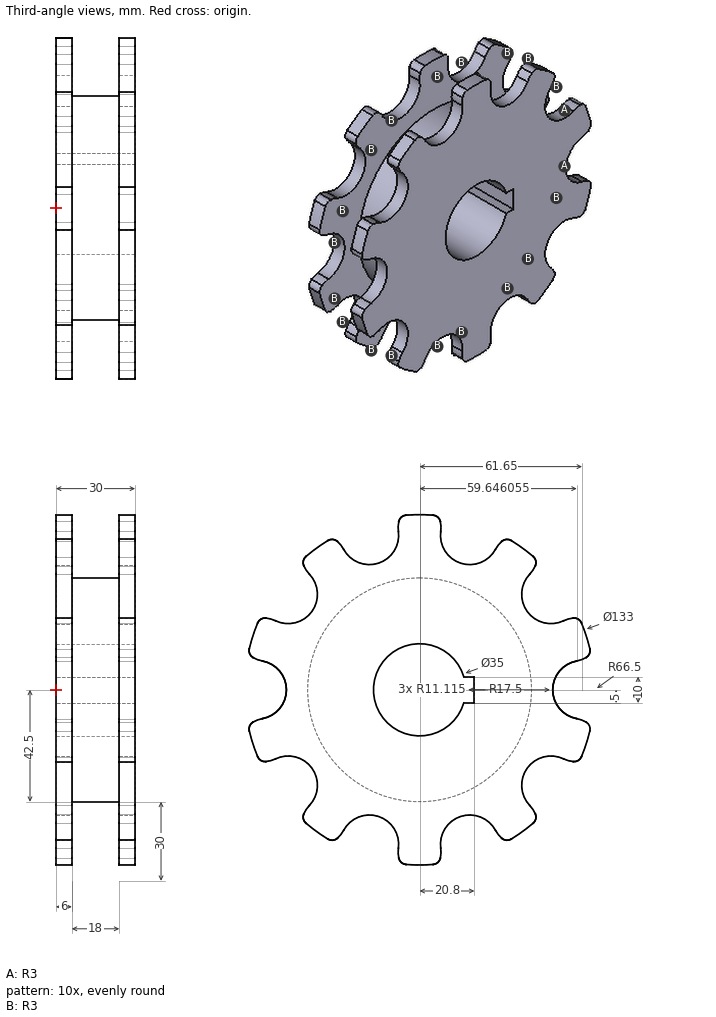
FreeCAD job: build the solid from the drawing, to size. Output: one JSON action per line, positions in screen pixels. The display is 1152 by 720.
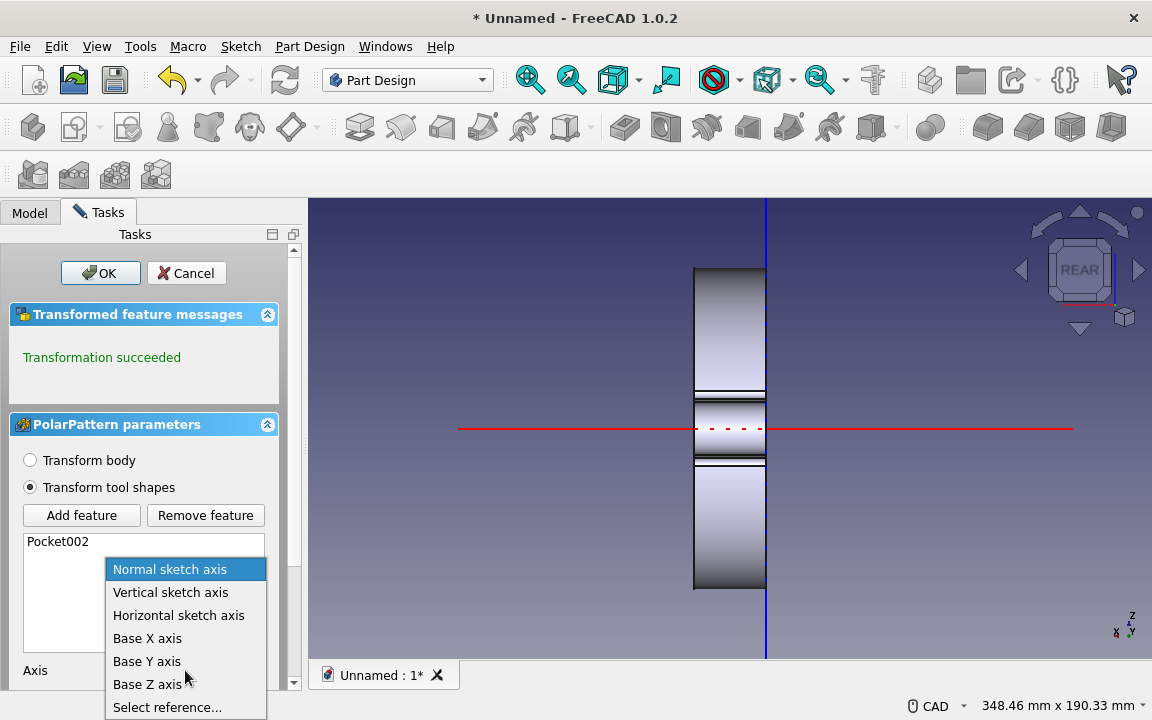
{"action": "left_click", "coordinate": [184, 638]}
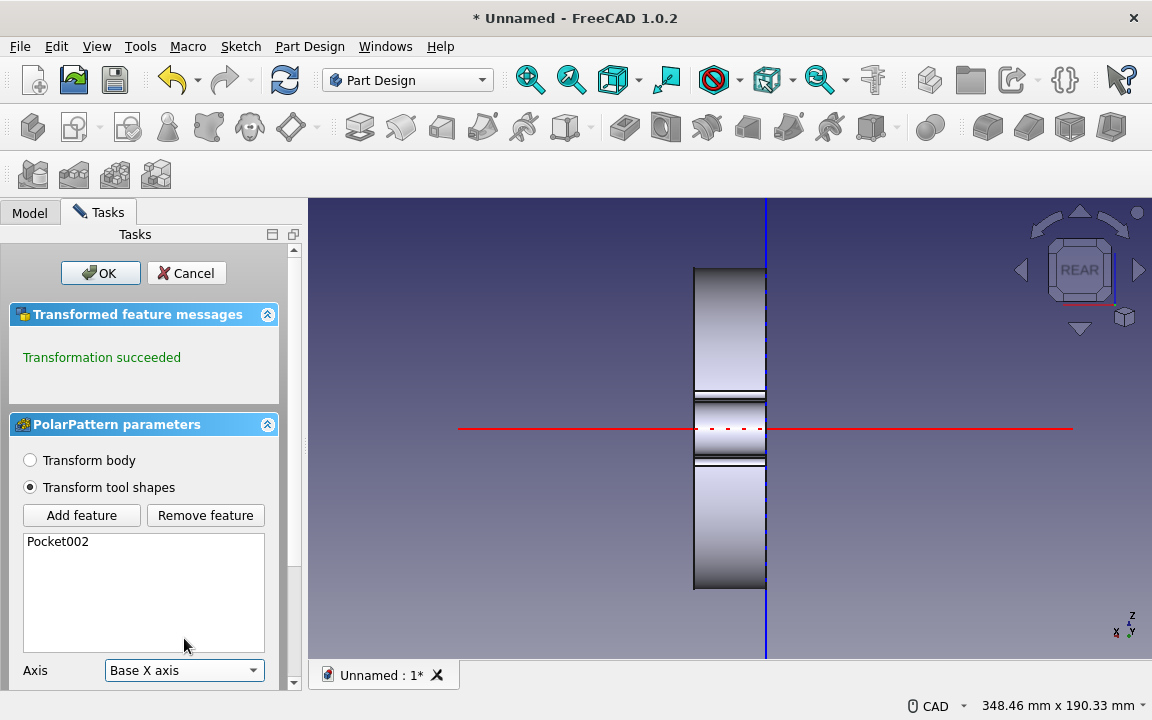
{"action": "scroll", "coordinate": [294, 467], "scroll_direction": "down", "scroll_amount": 3}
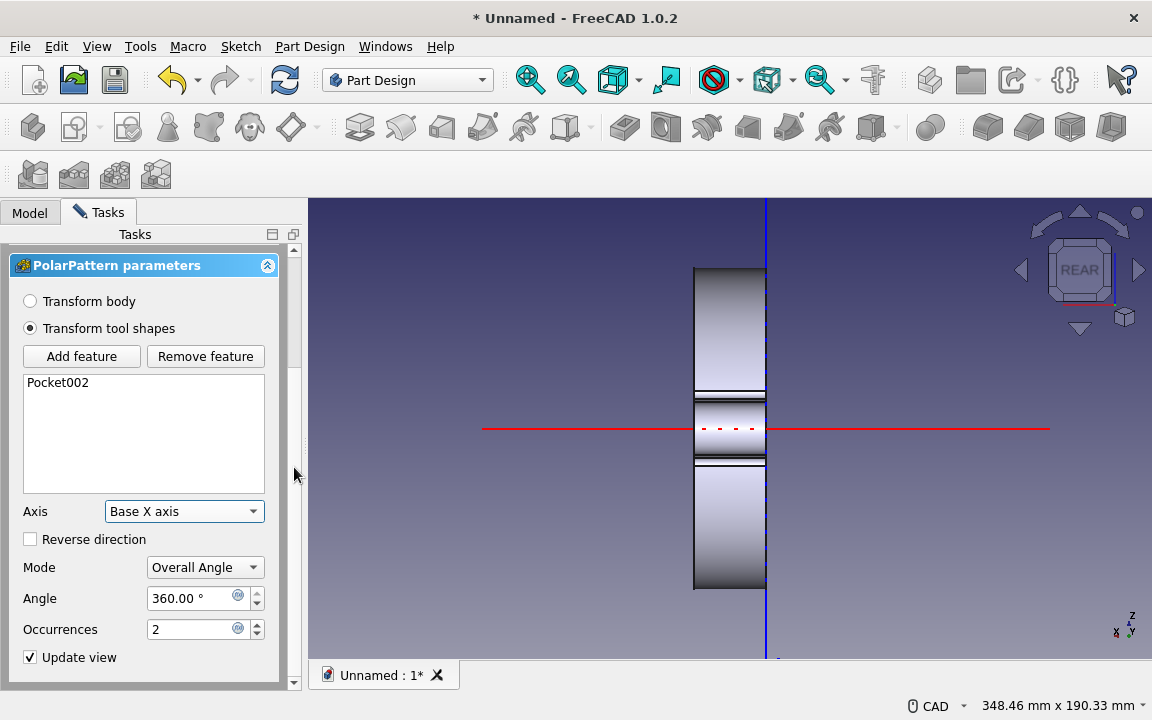
{"action": "triple_click", "coordinate": [199, 630]}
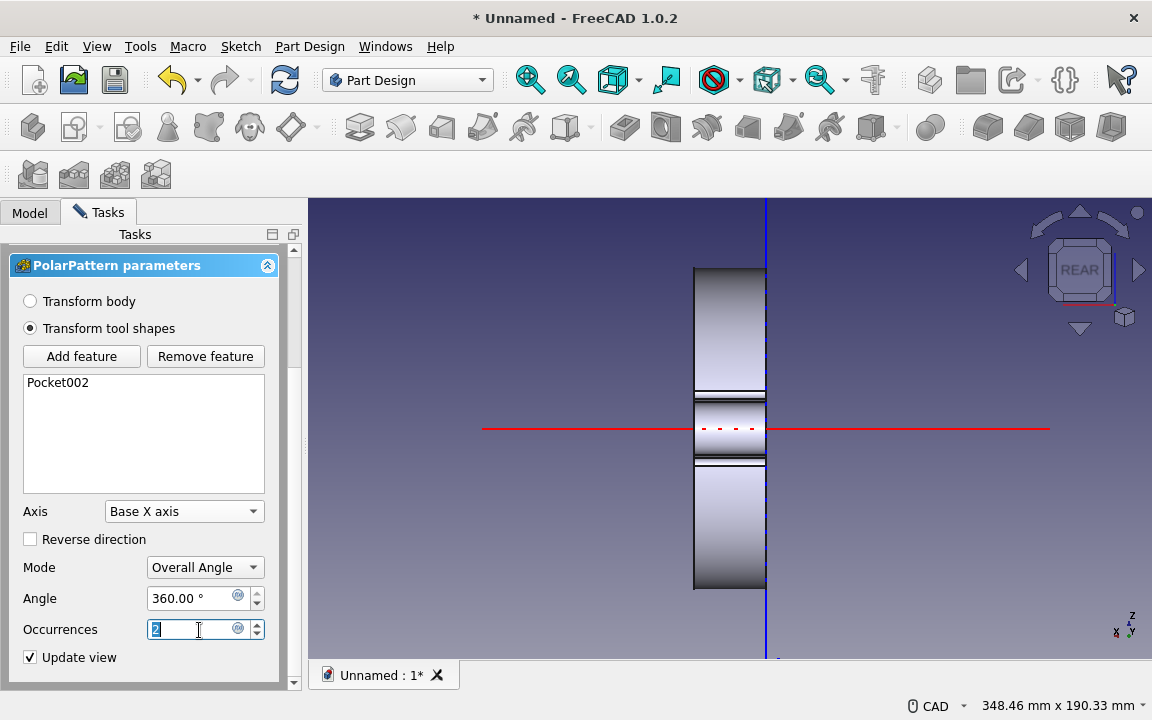
{"action": "type", "text": "10"}
{"action": "key", "text": "Tab"}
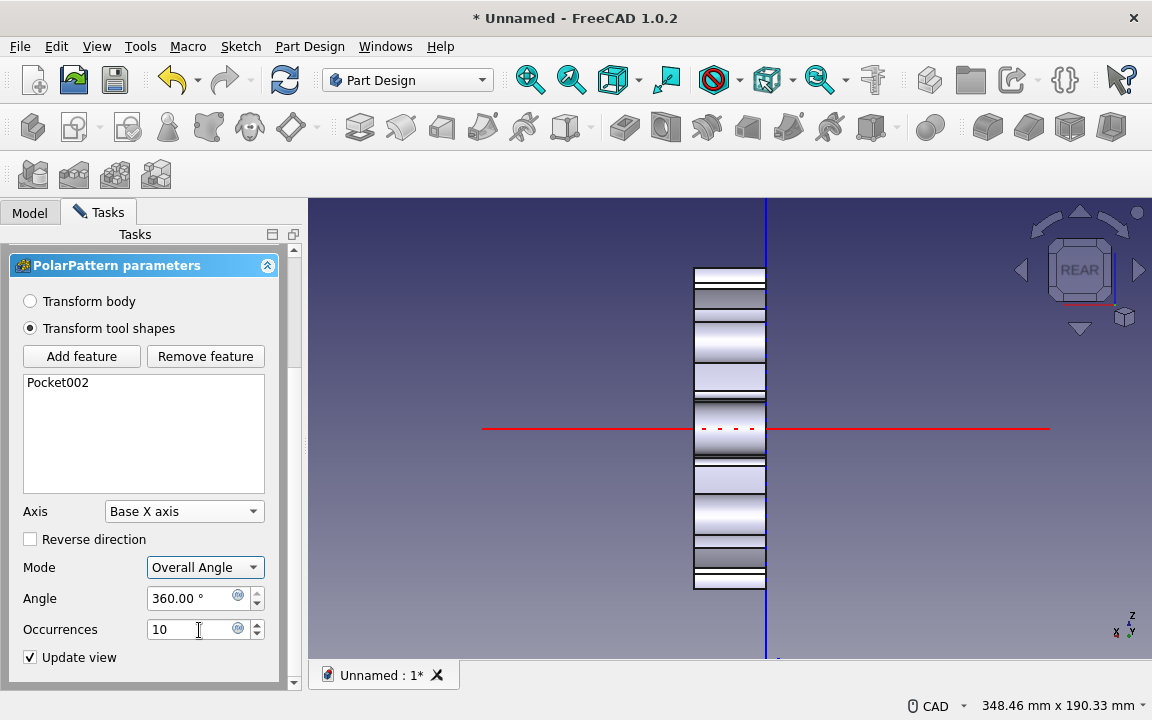
{"action": "scroll", "coordinate": [294, 467], "scroll_direction": "up", "scroll_amount": 4}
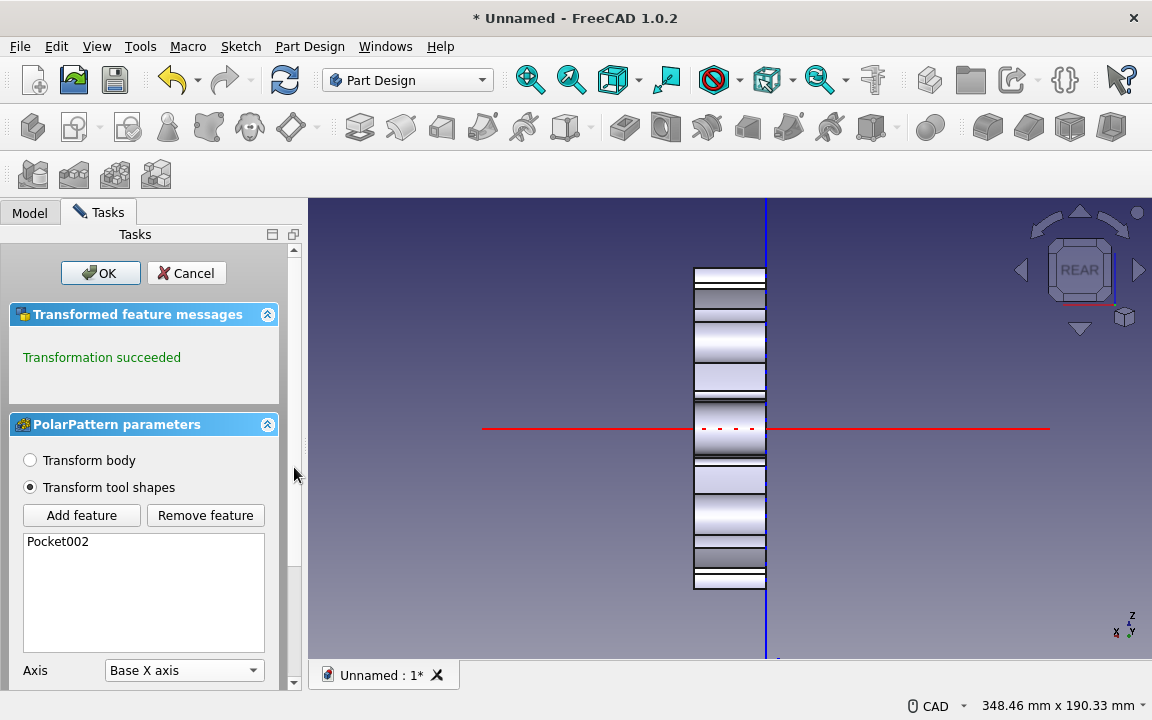
{"action": "left_click", "coordinate": [101, 273]}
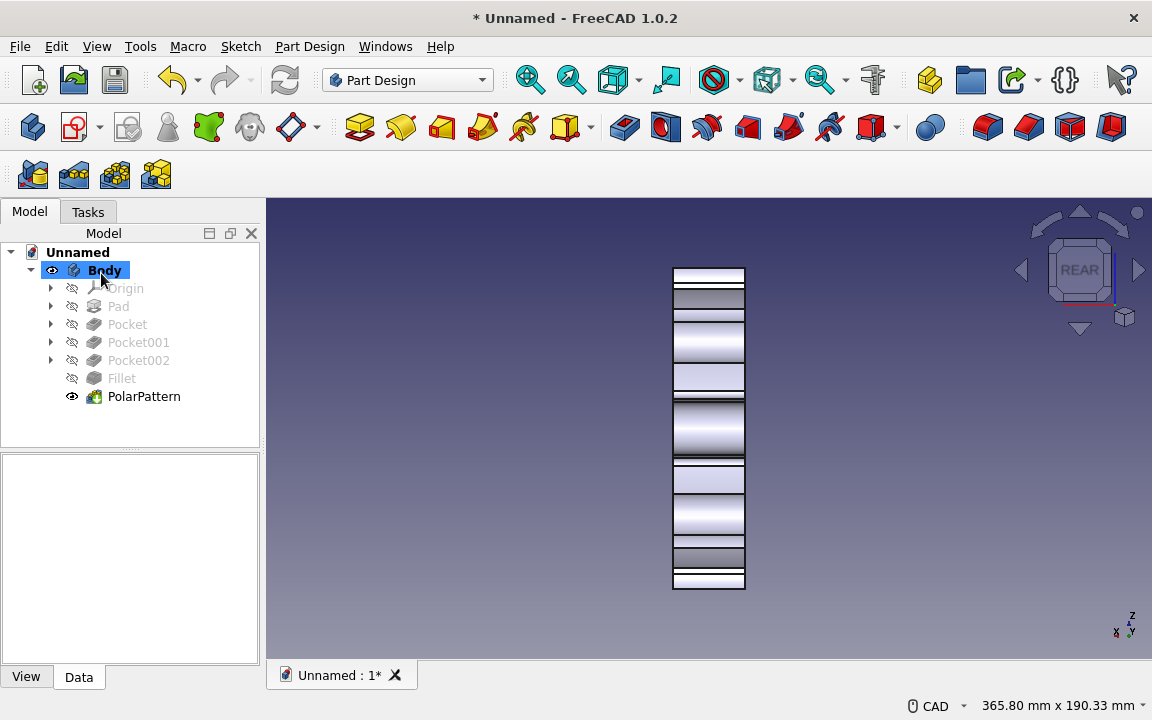
{"action": "left_click", "coordinate": [709, 308]}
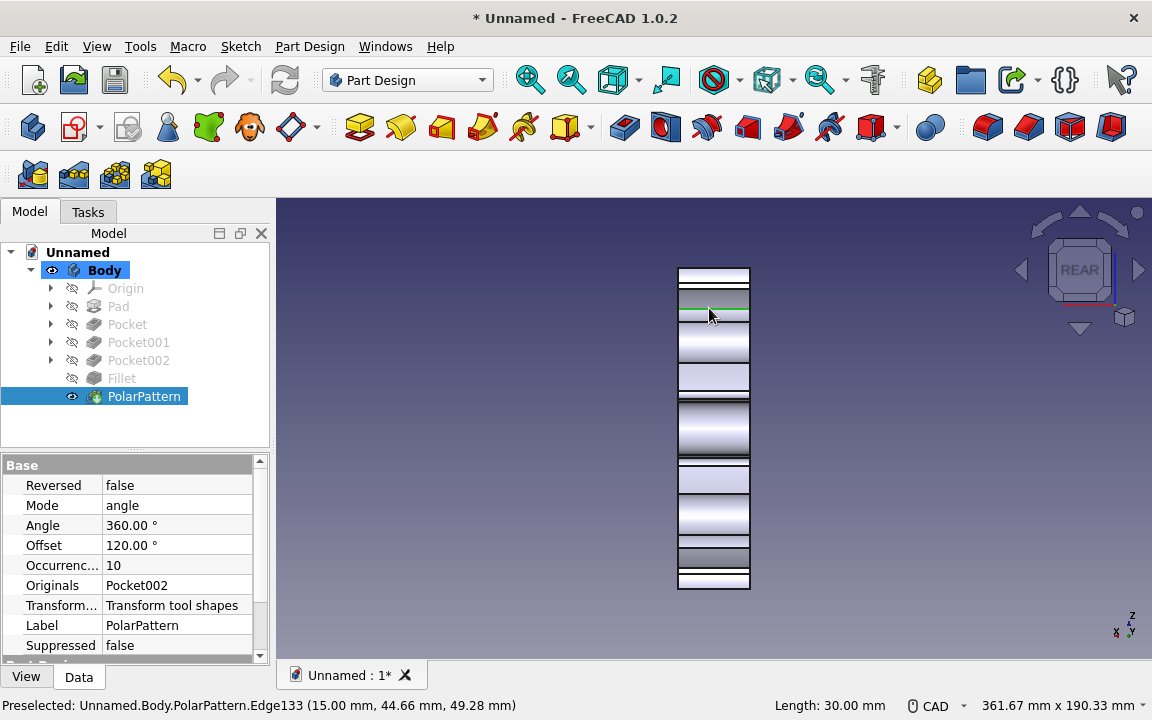
{"action": "left_click", "coordinate": [714, 547], "text": "ctrl"}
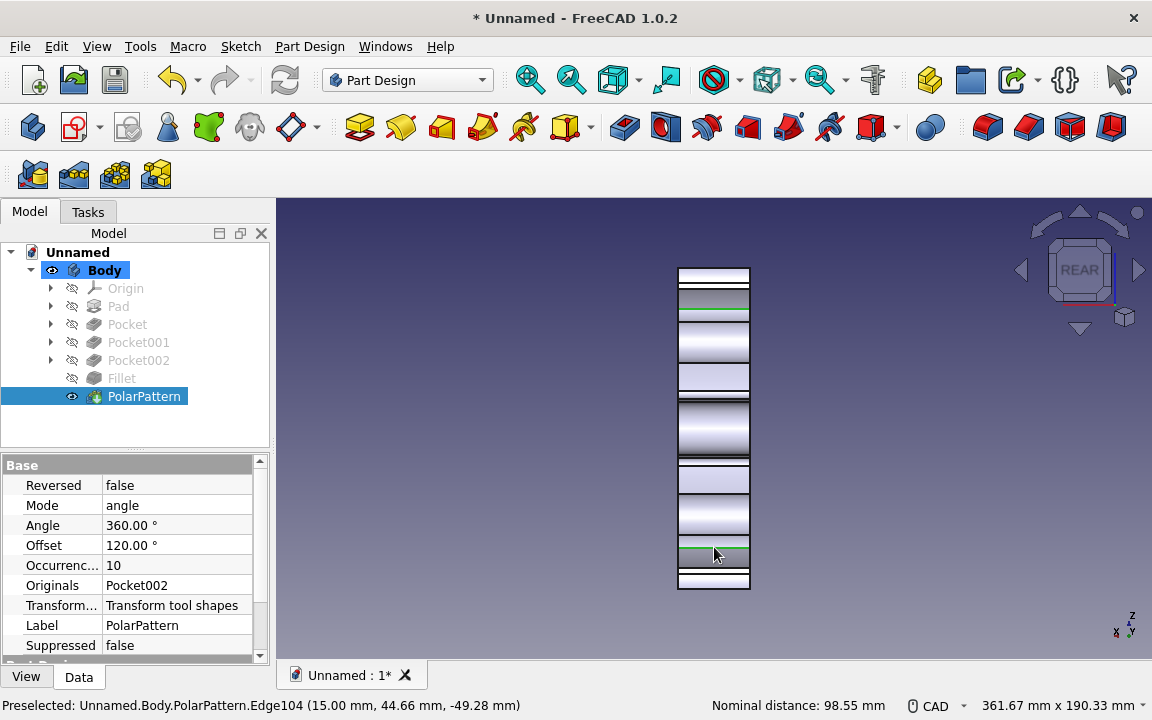
{"action": "key", "text": "0"}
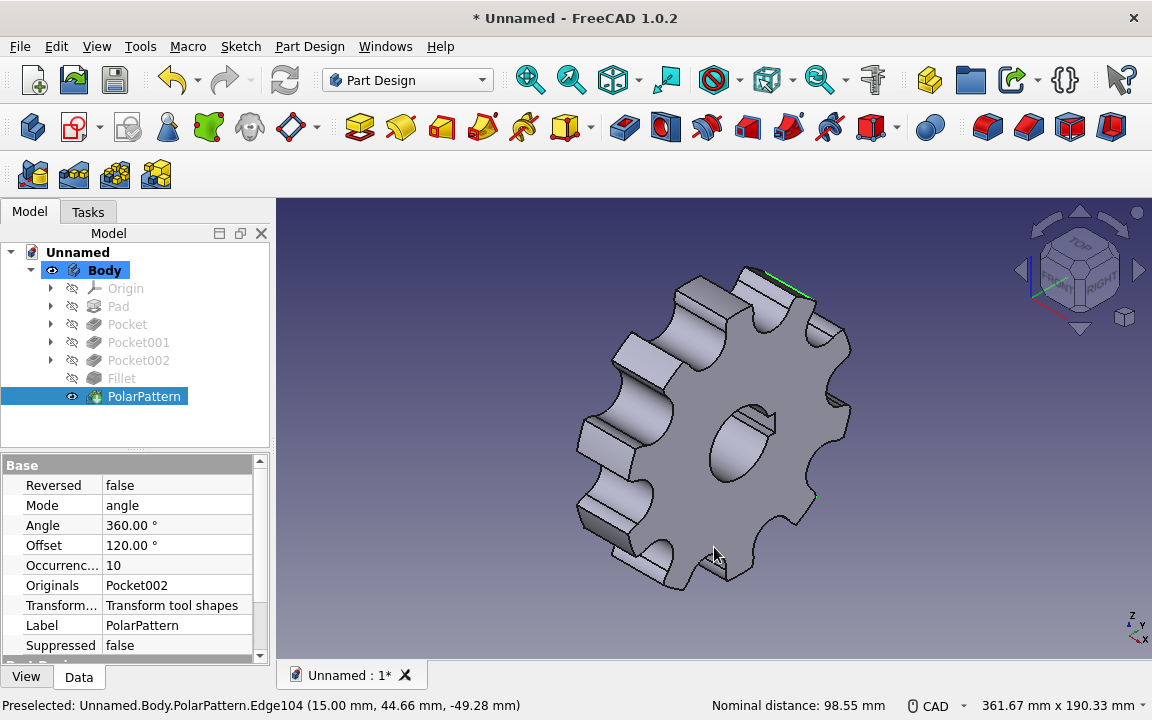
{"action": "left_click", "coordinate": [702, 304], "text": "ctrl"}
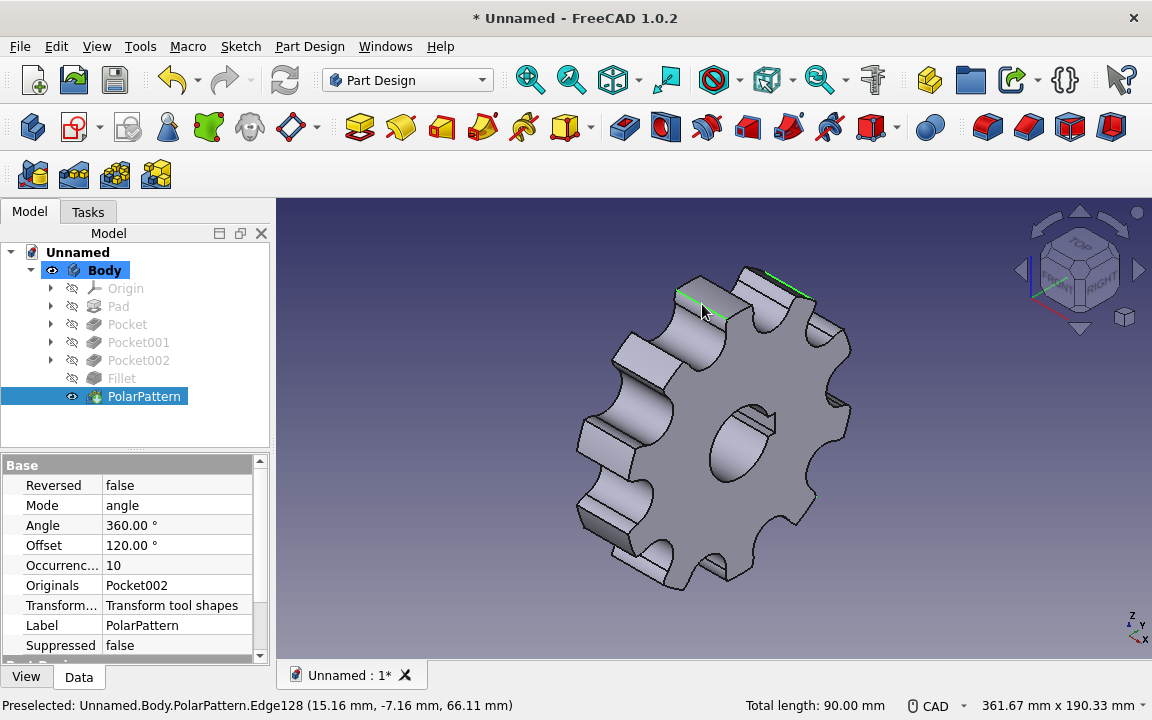
{"action": "left_click", "coordinate": [610, 434], "text": "ctrl"}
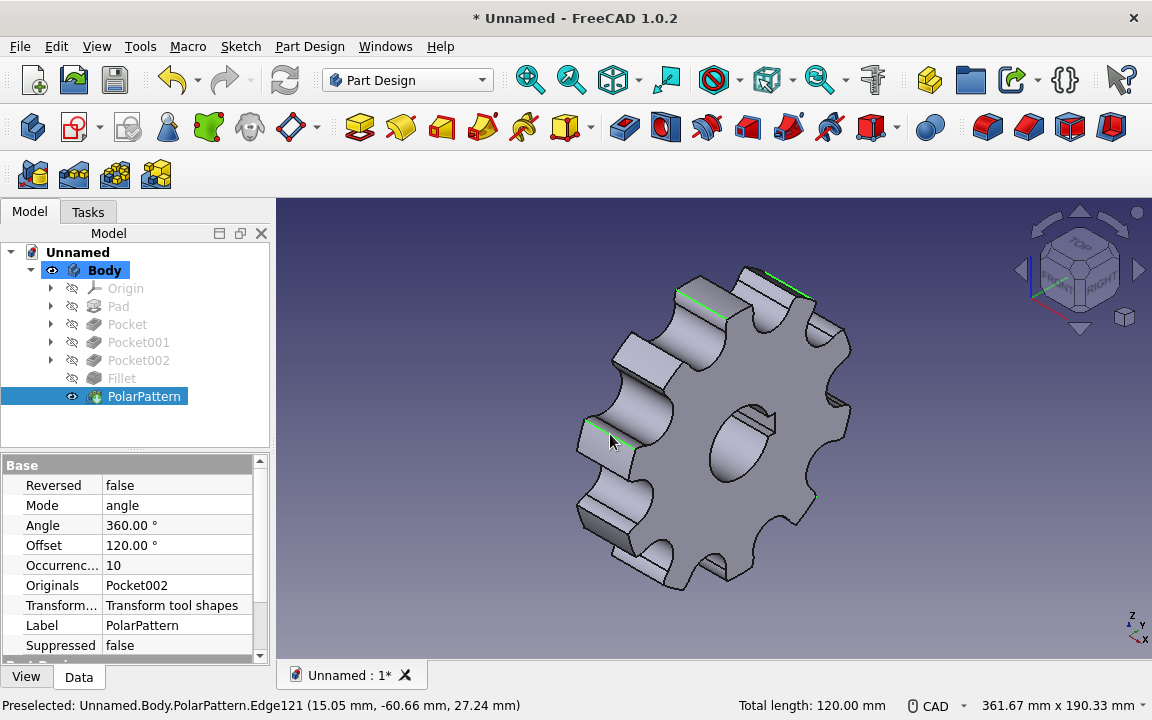
{"action": "left_click", "coordinate": [638, 374], "text": "ctrl"}